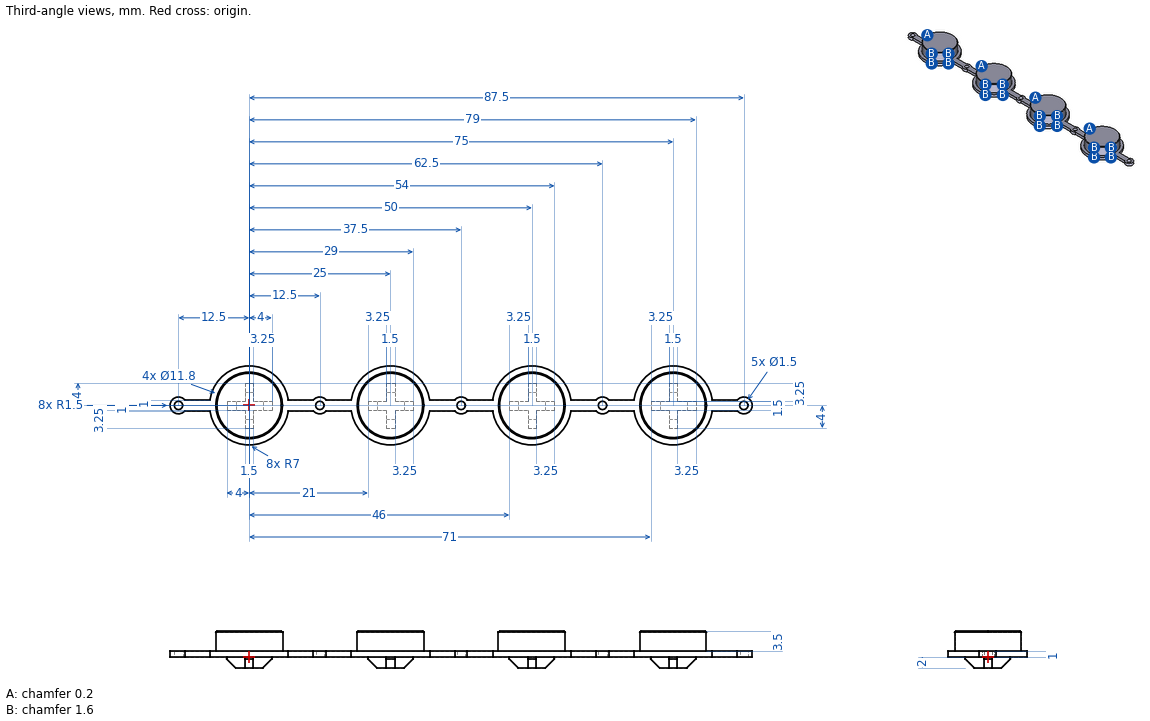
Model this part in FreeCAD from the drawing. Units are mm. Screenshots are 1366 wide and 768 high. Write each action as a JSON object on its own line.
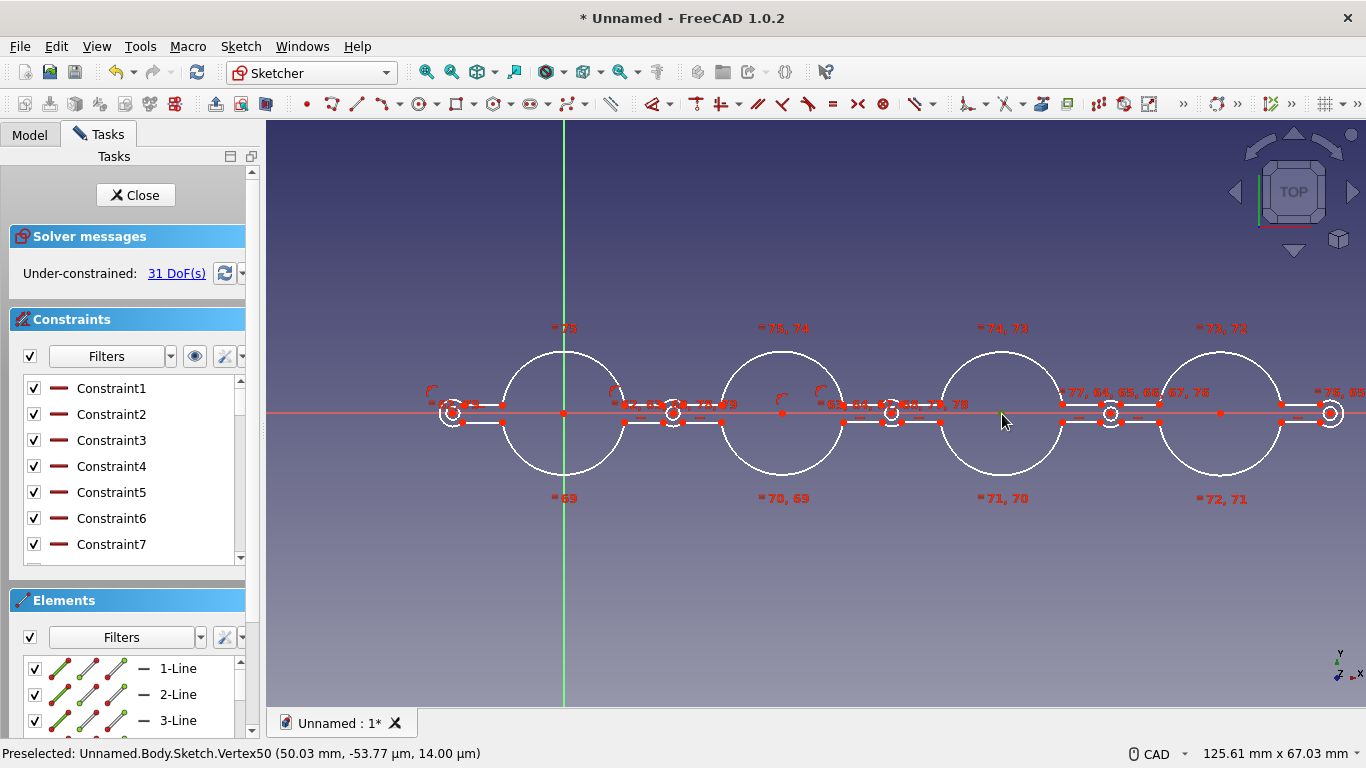
{"action": "left_click", "coordinate": [359, 413]}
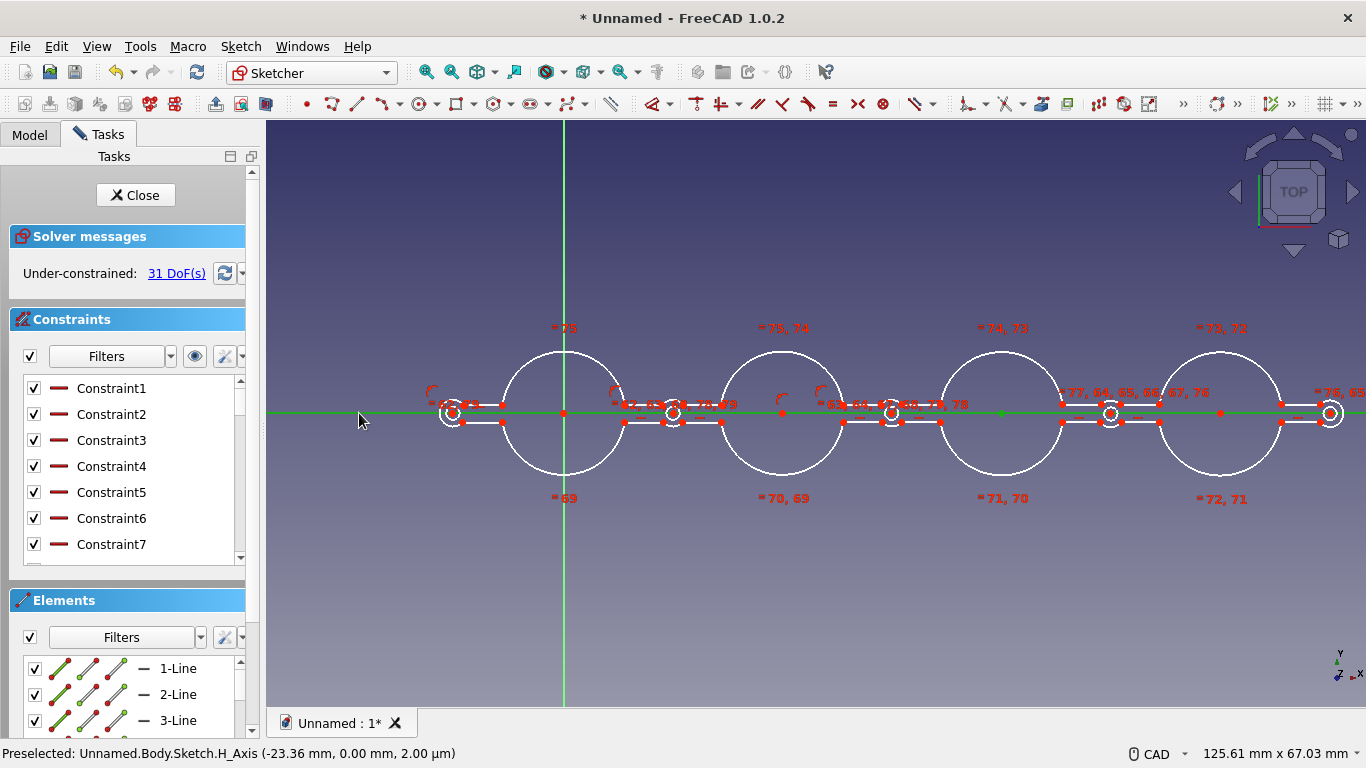
{"action": "left_click", "coordinate": [696, 104]}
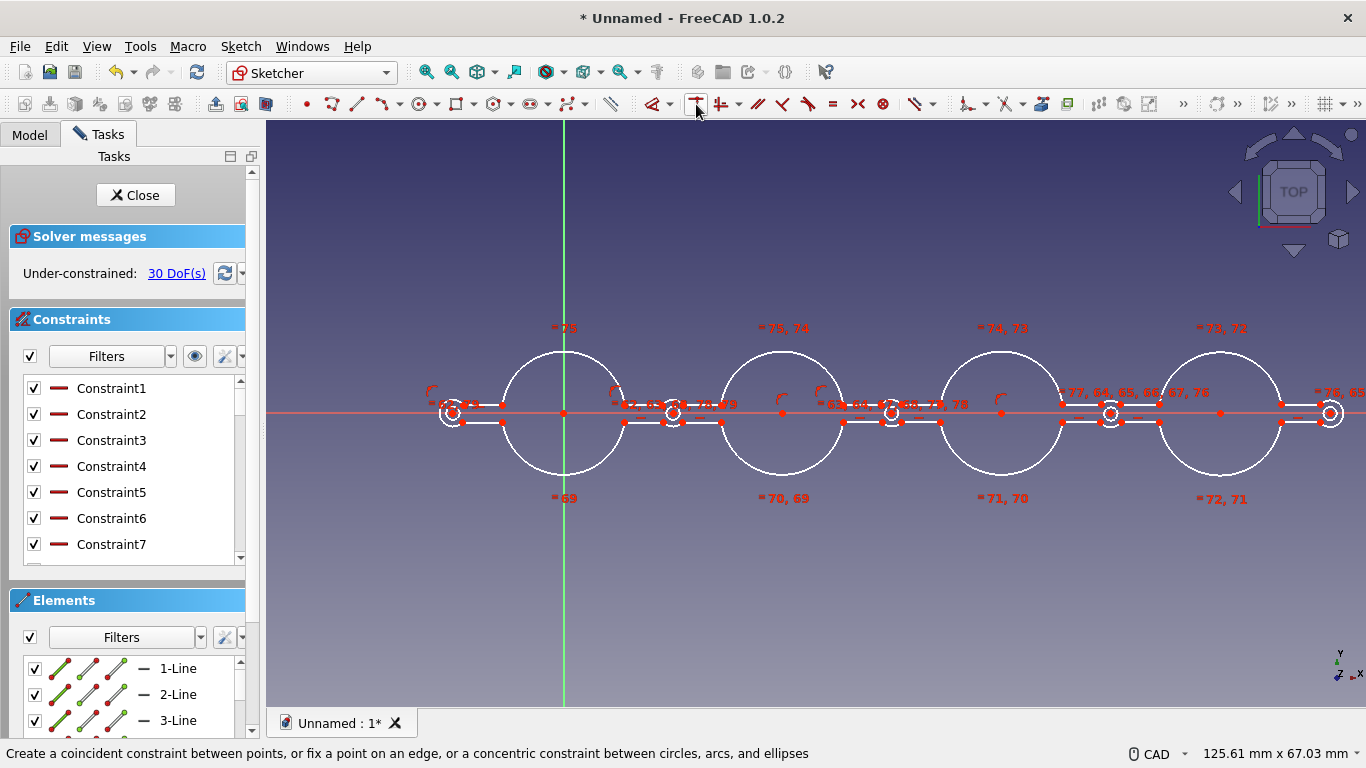
{"action": "left_click", "coordinate": [1111, 414]}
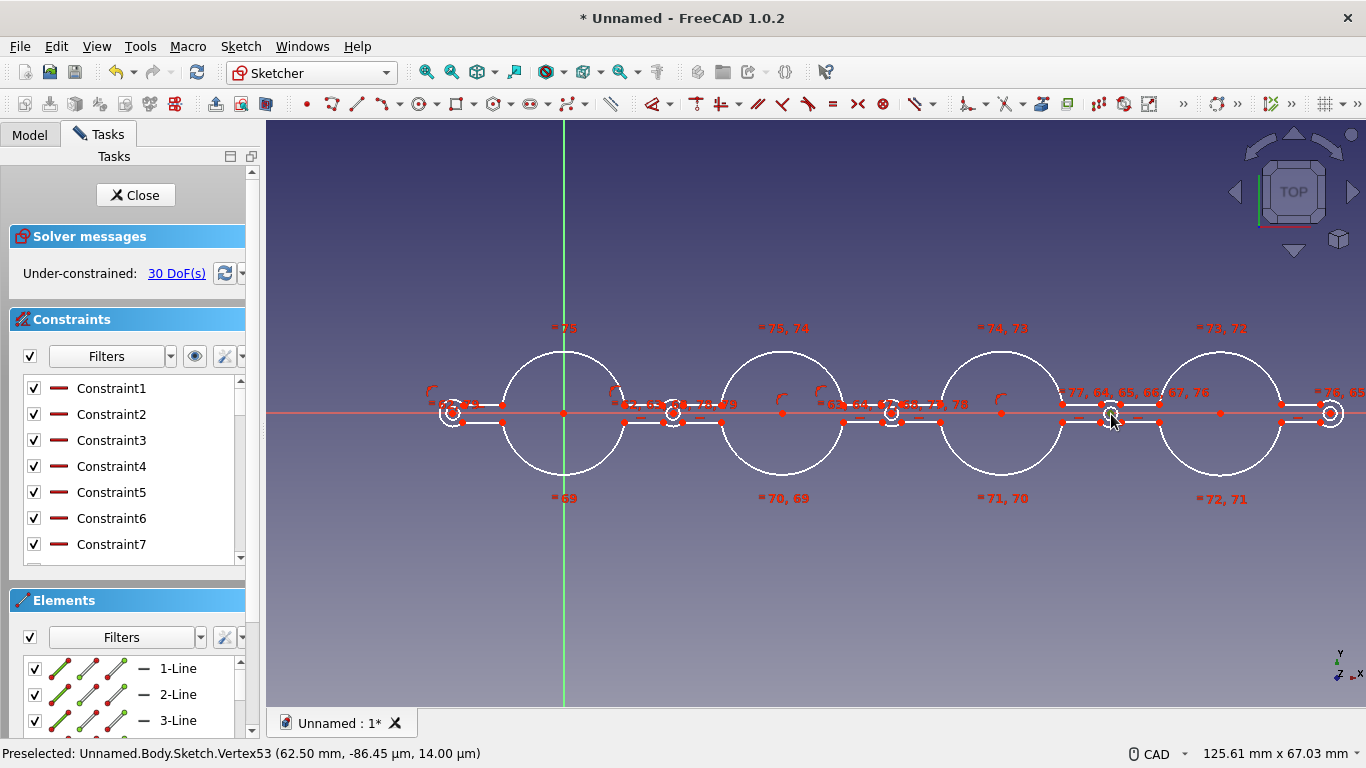
{"action": "left_click", "coordinate": [359, 413]}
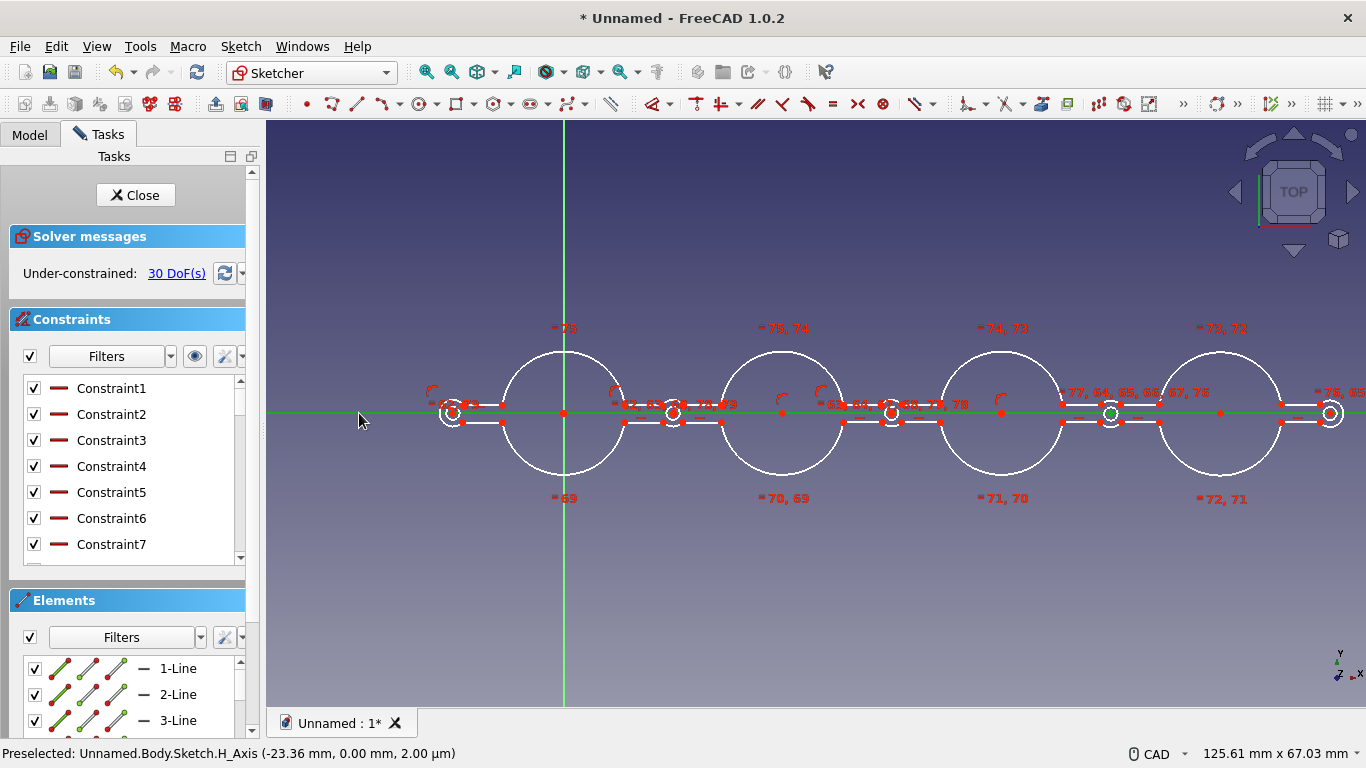
{"action": "key", "text": "c"}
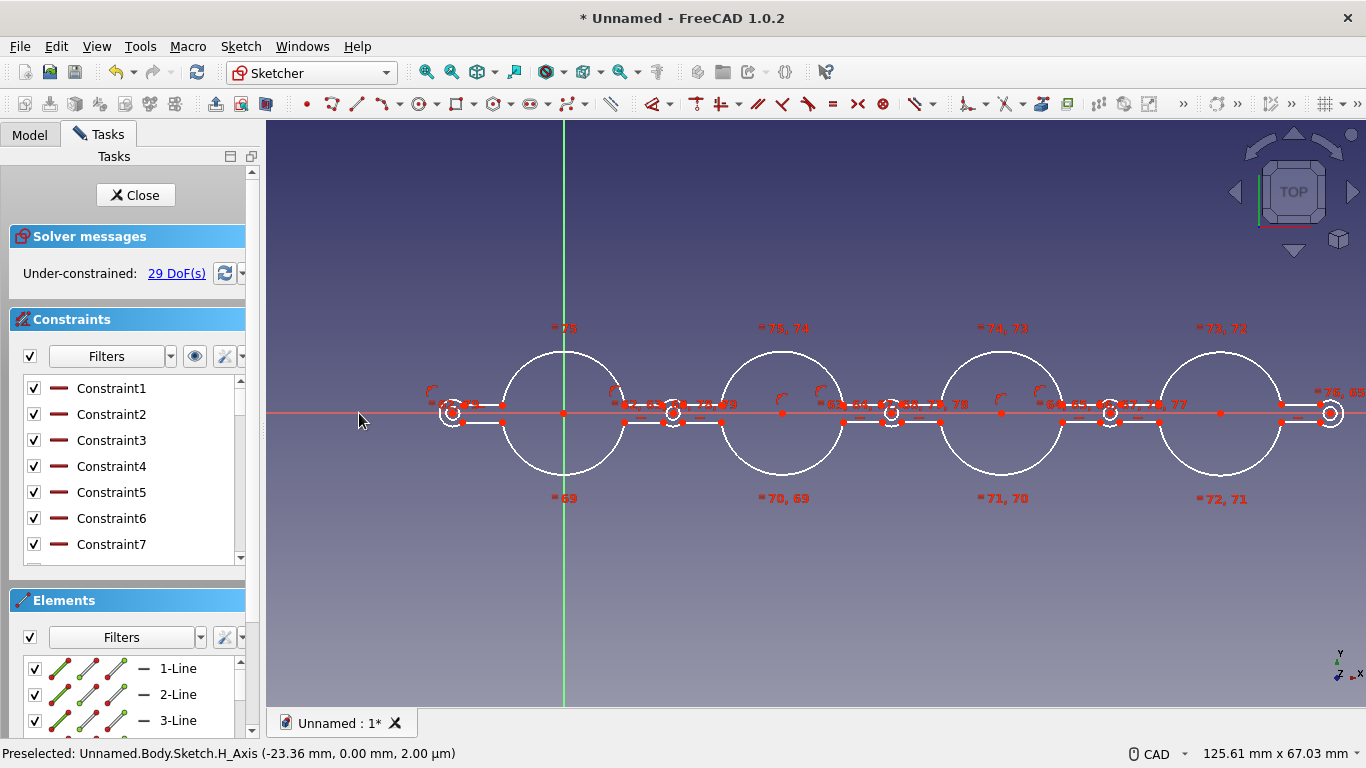
{"action": "scroll", "coordinate": [454, 414], "scroll_direction": "down", "scroll_amount": 2}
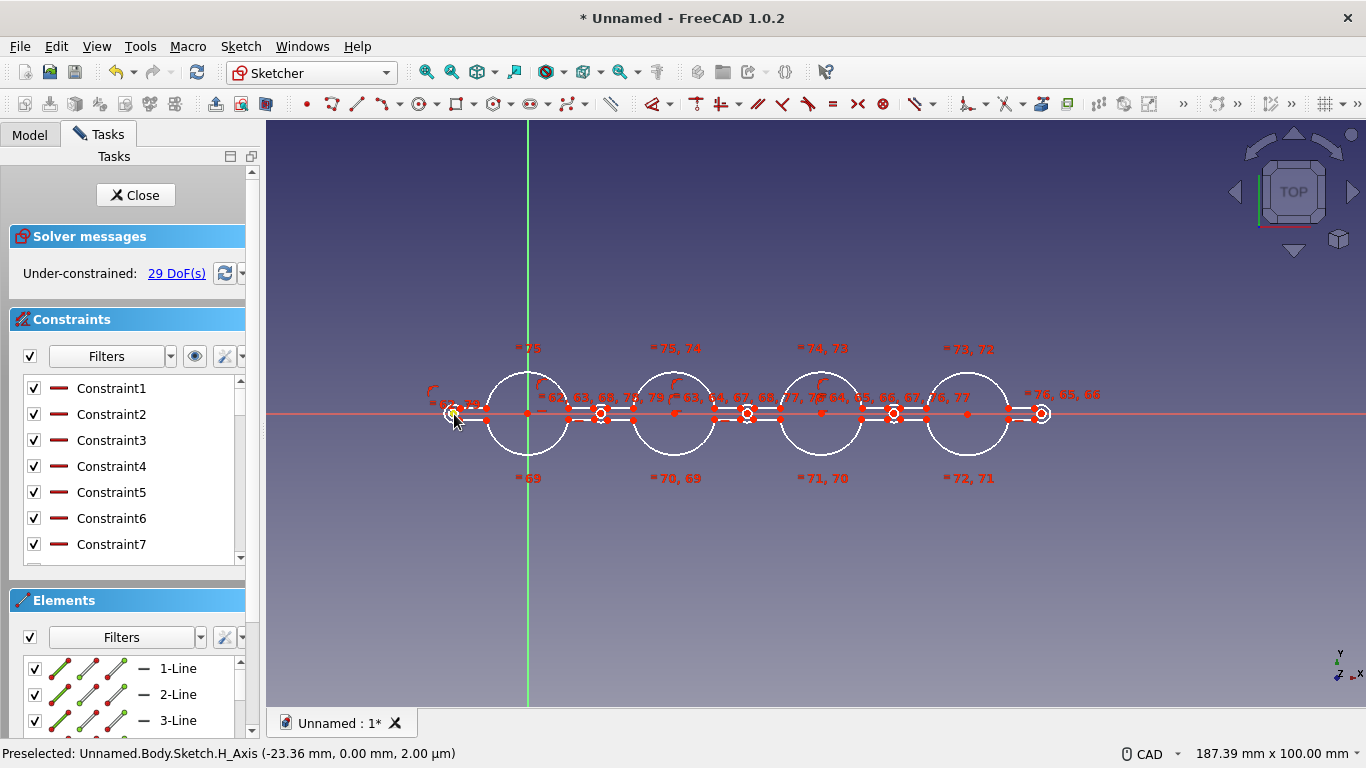
{"action": "left_click", "coordinate": [968, 414]}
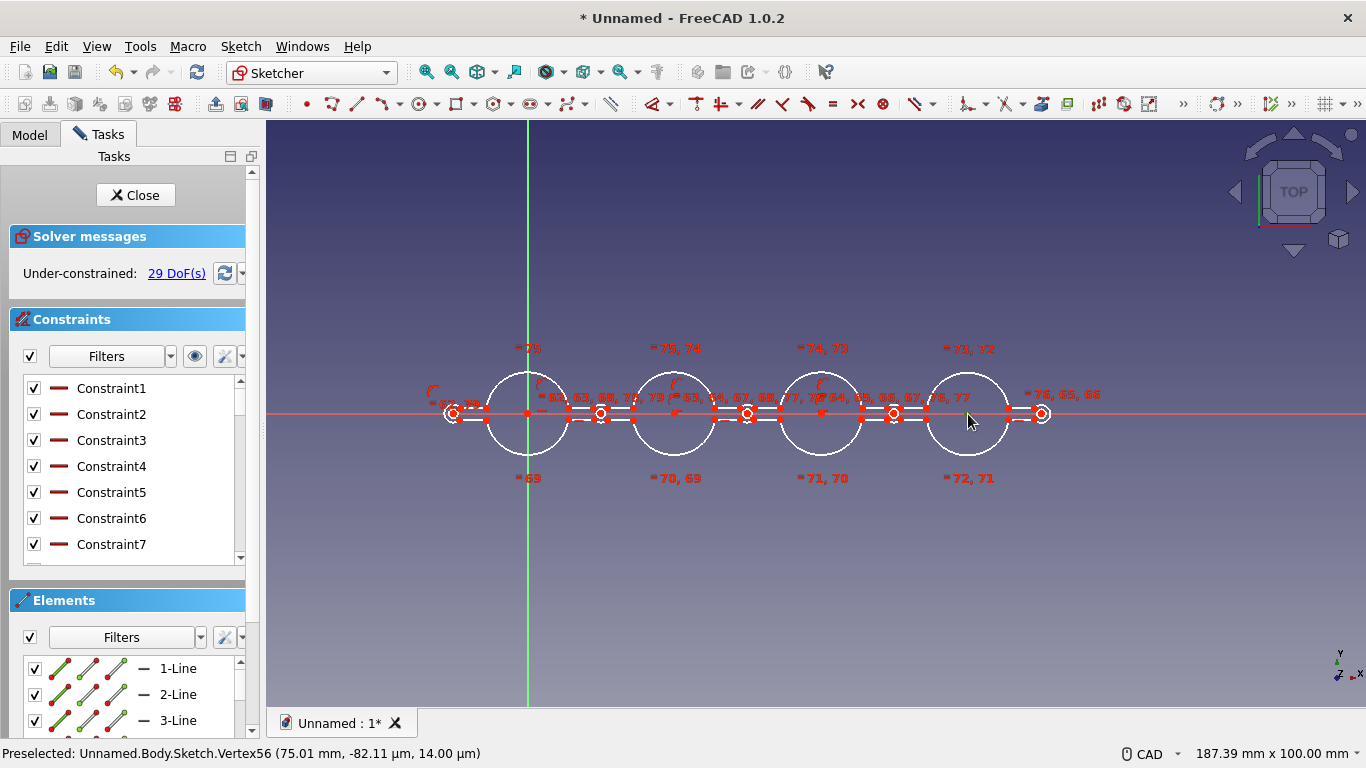
{"action": "left_click", "coordinate": [359, 414]}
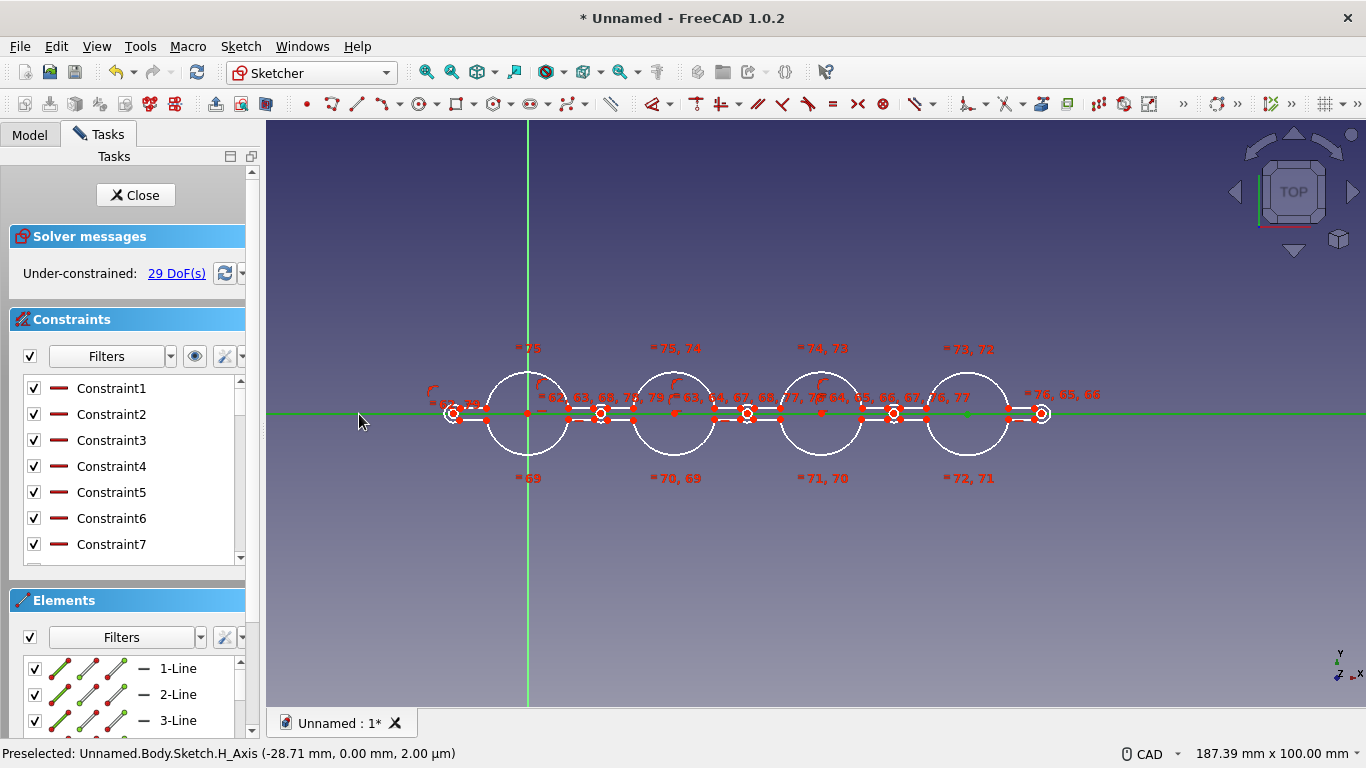
{"action": "left_click", "coordinate": [696, 104]}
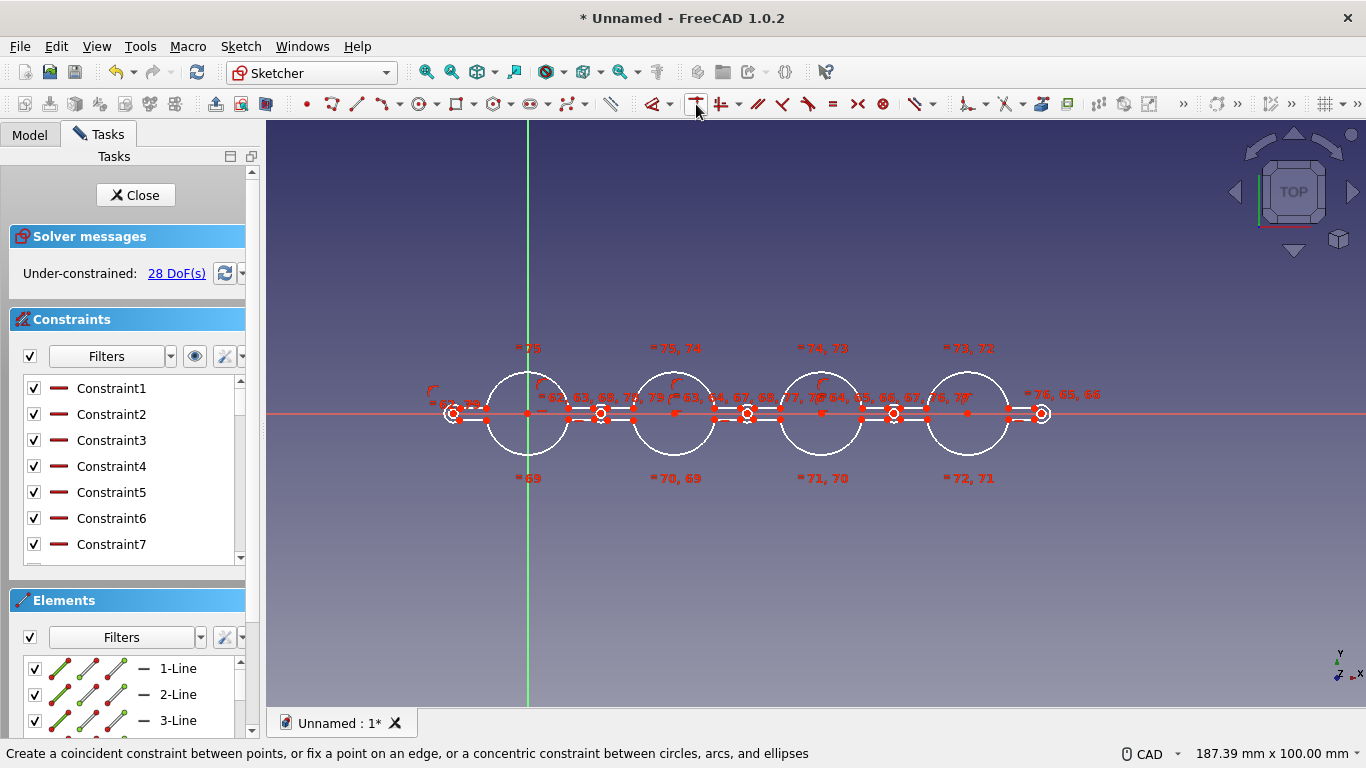
{"action": "scroll", "coordinate": [1041, 414], "scroll_direction": "up", "scroll_amount": 2}